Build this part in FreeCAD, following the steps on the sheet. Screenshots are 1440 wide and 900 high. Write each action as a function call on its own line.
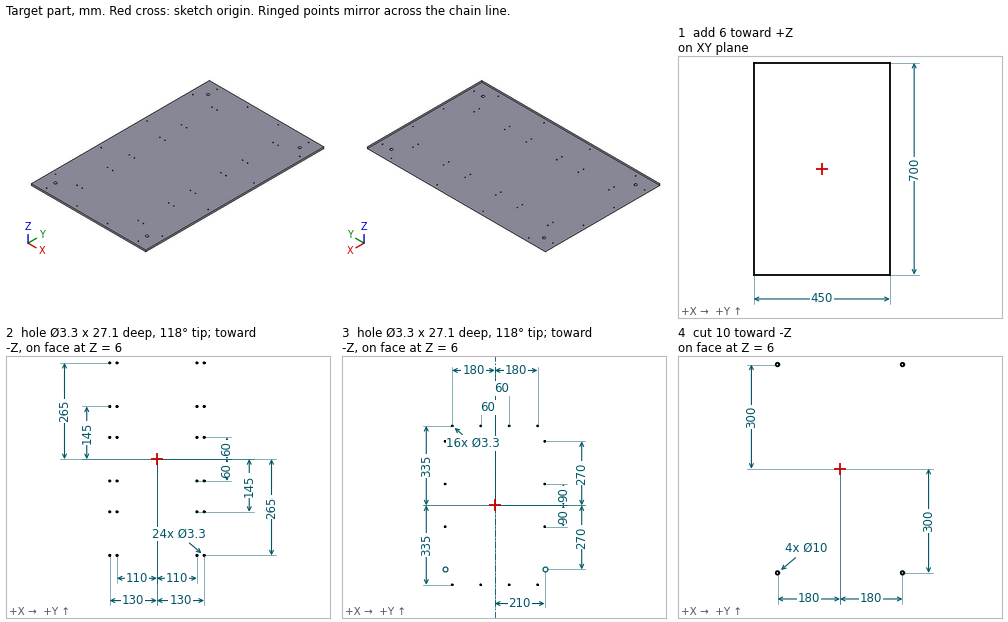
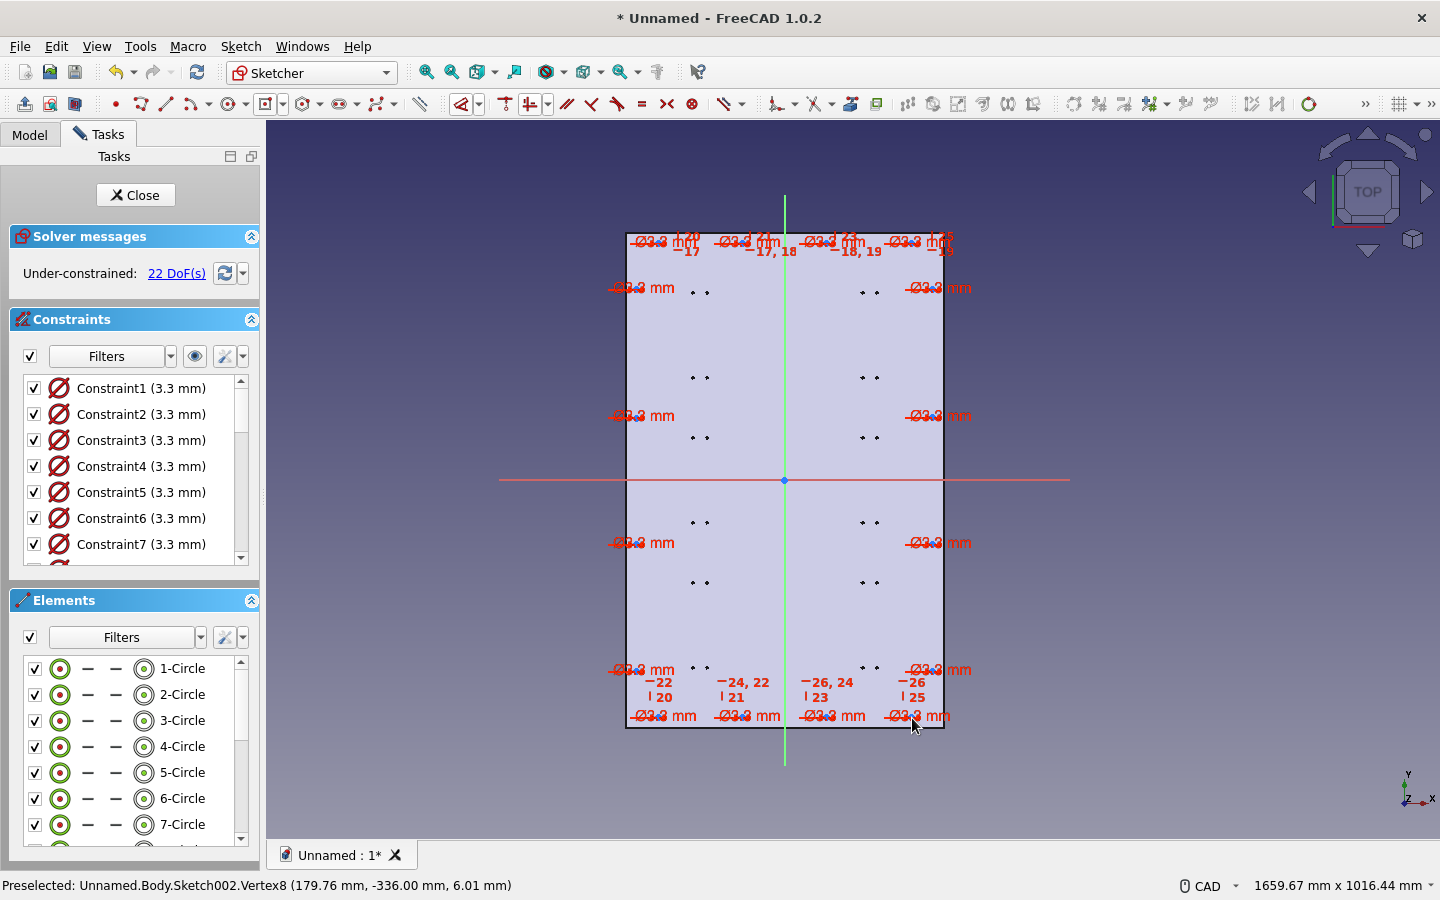
click(933, 672)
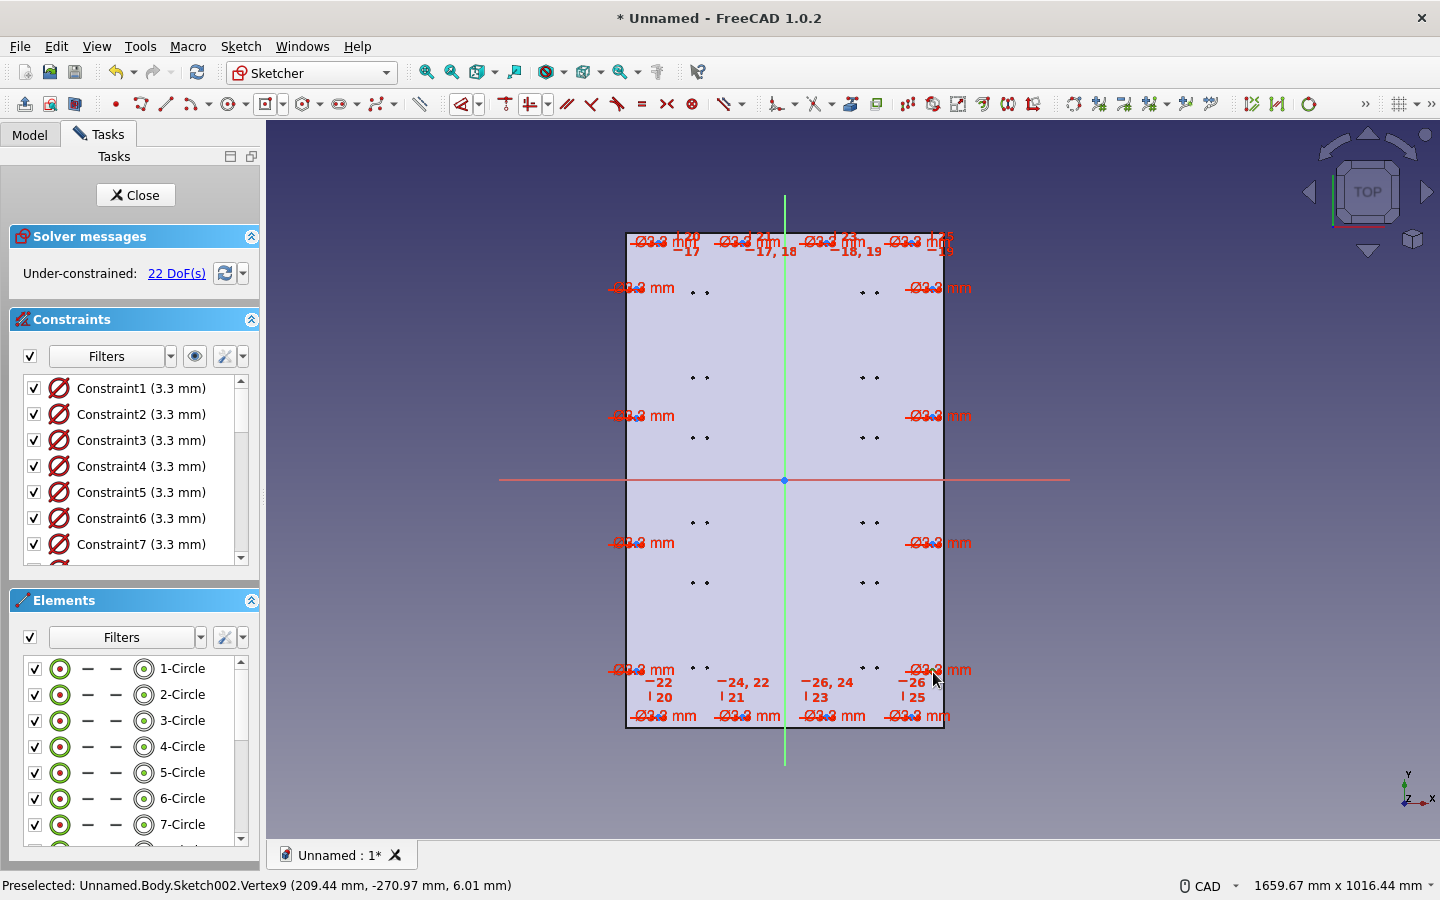
click(933, 545)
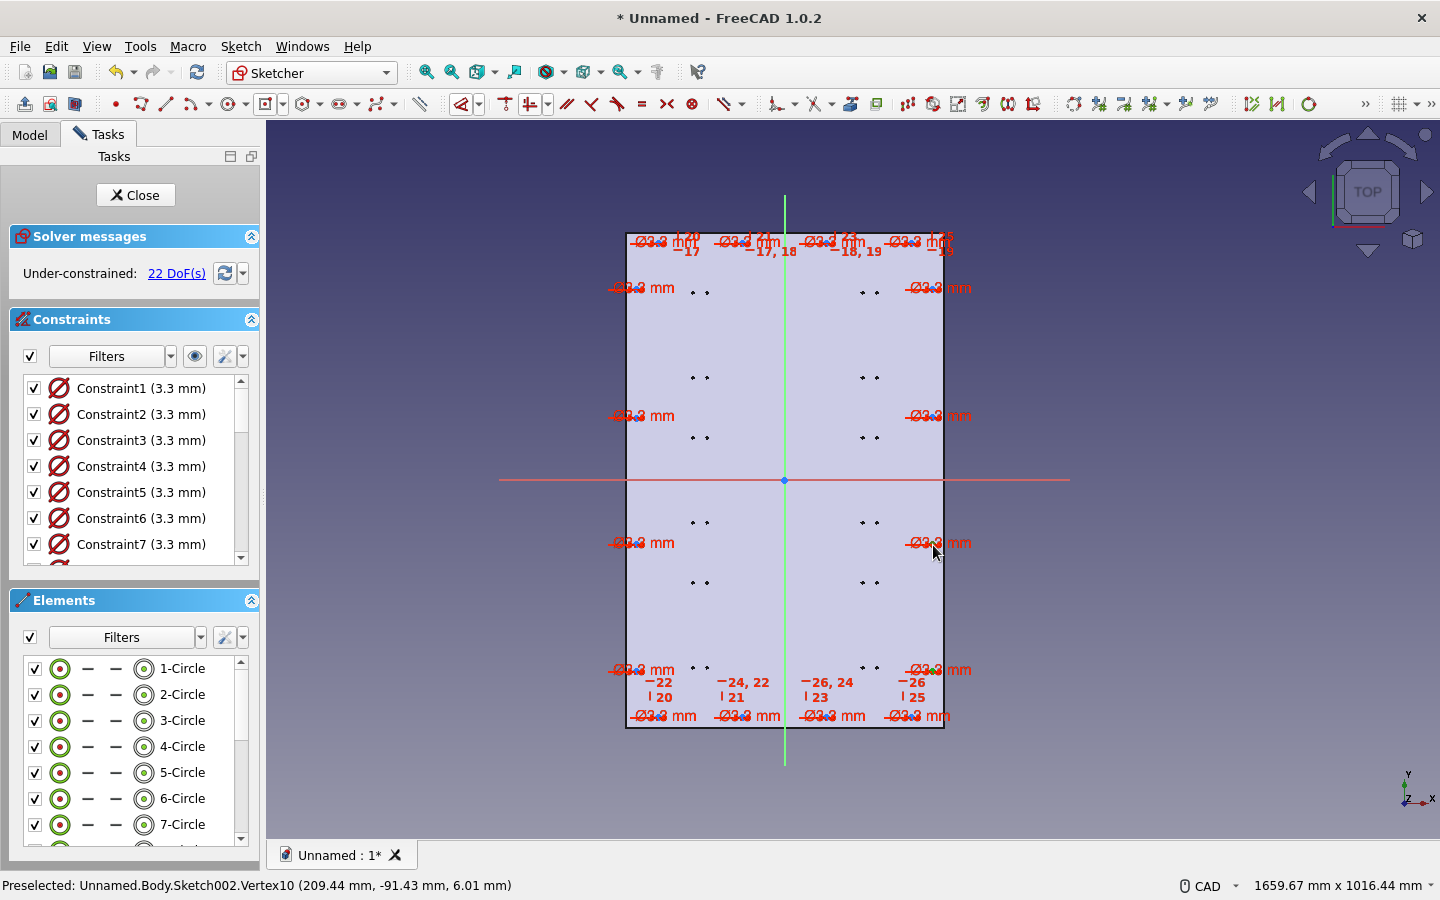
click(548, 104)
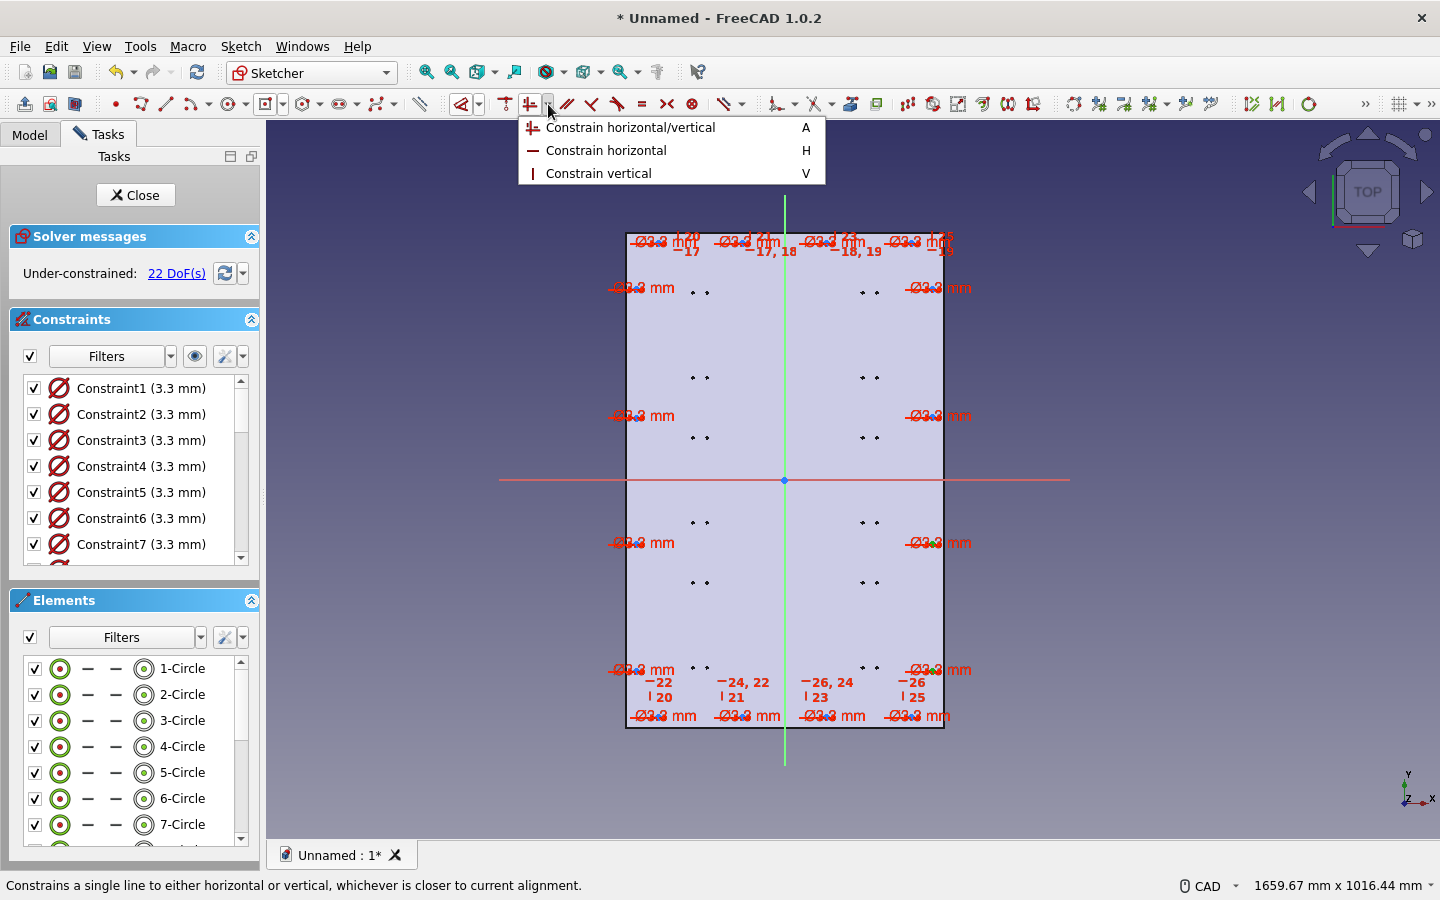
click(672, 174)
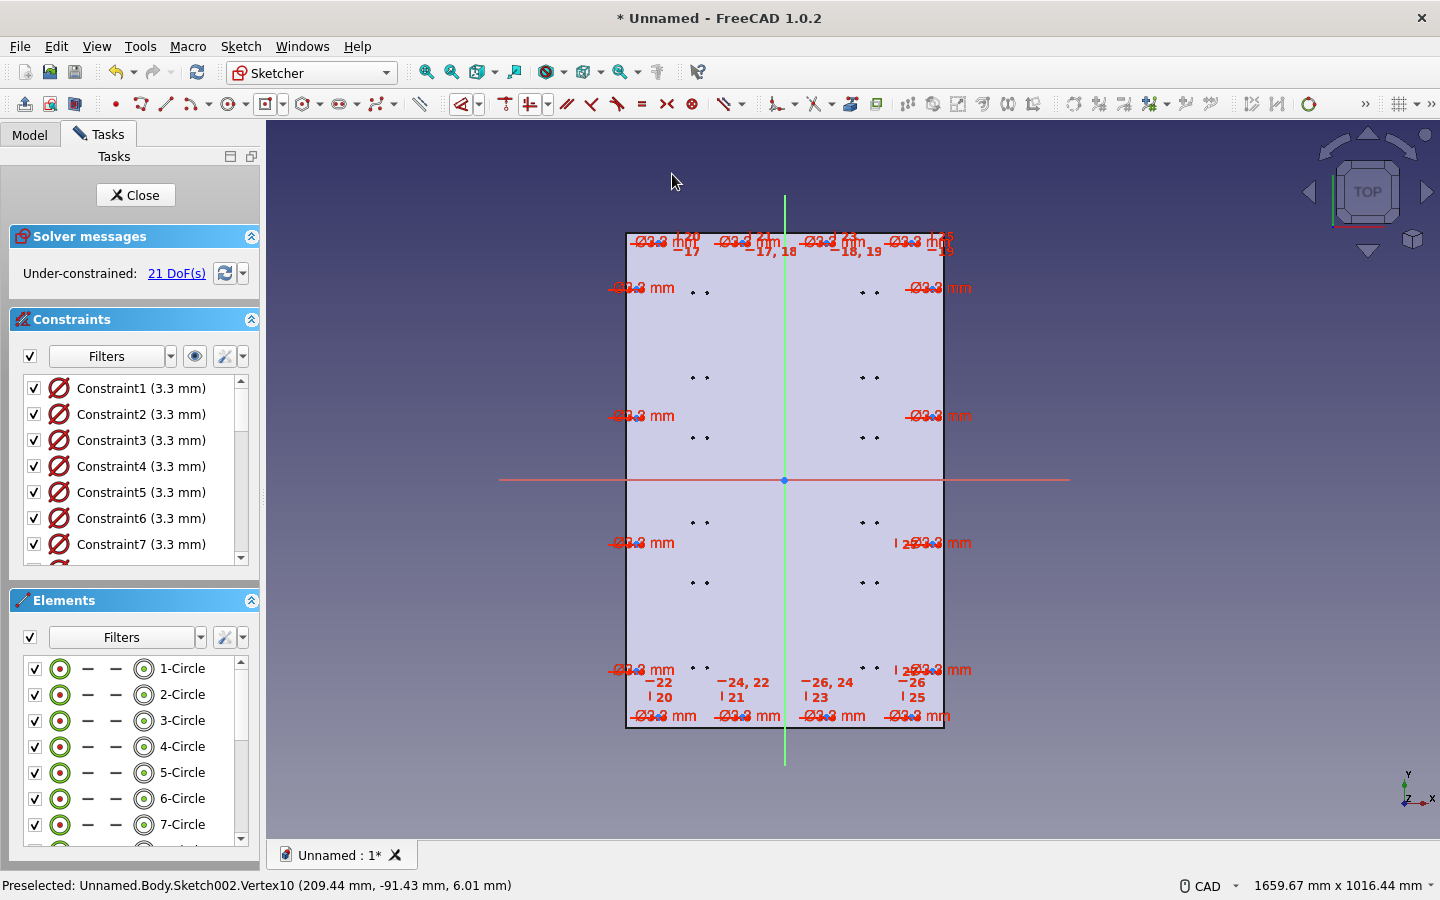
click(933, 545)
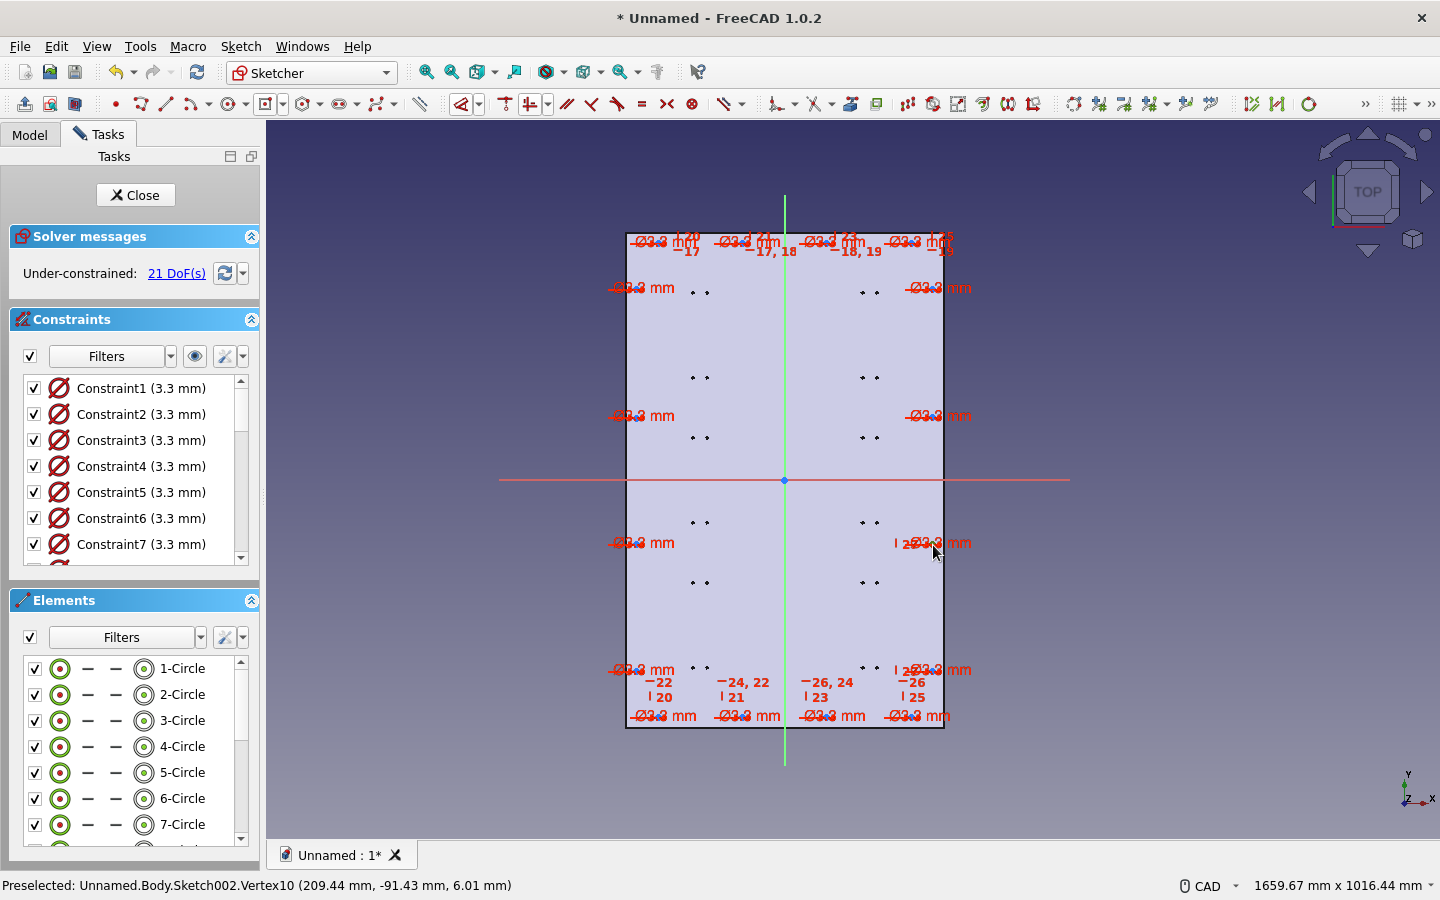
click(933, 418)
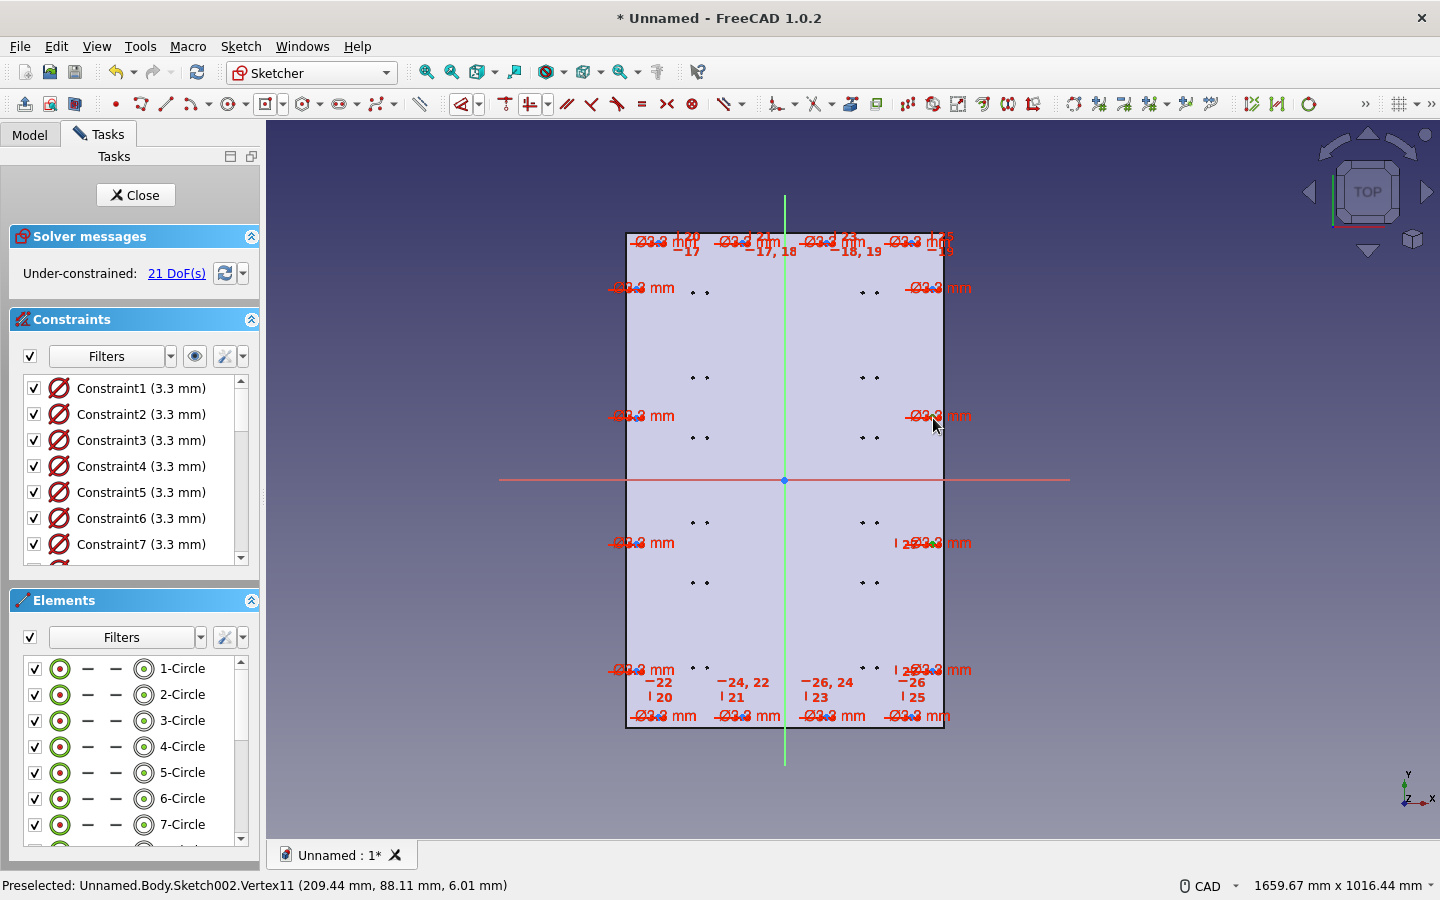
key(v)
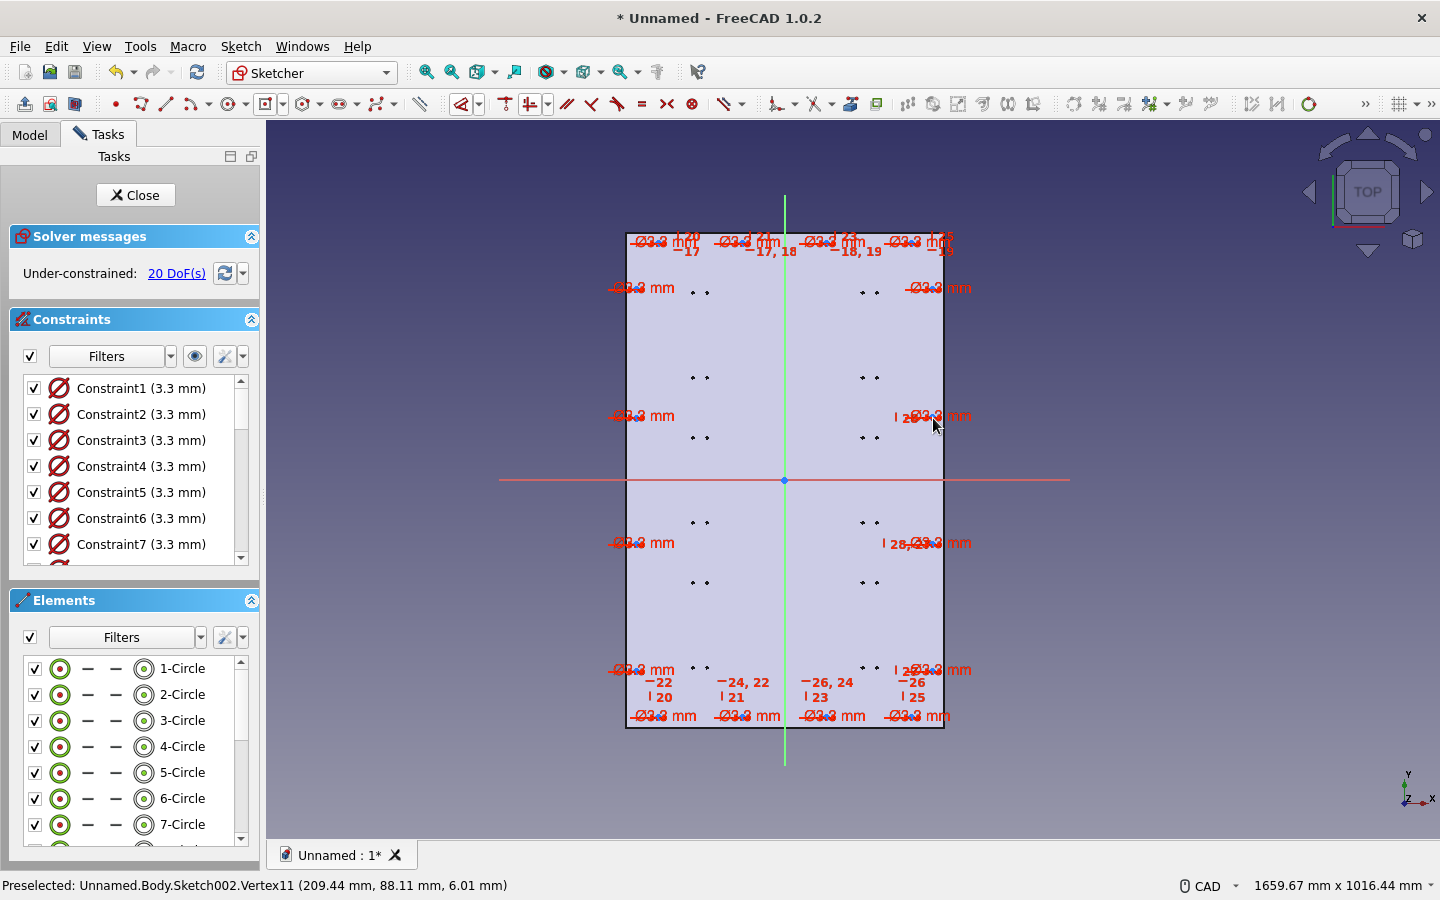
click(933, 418)